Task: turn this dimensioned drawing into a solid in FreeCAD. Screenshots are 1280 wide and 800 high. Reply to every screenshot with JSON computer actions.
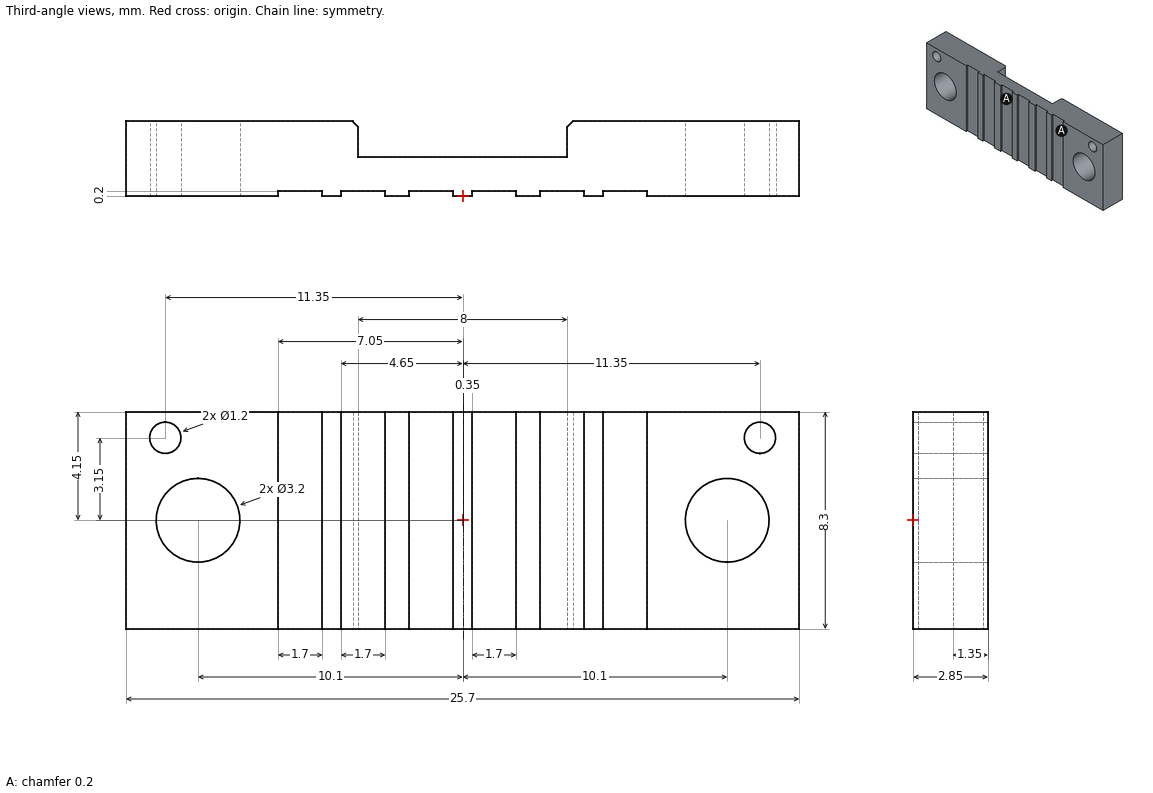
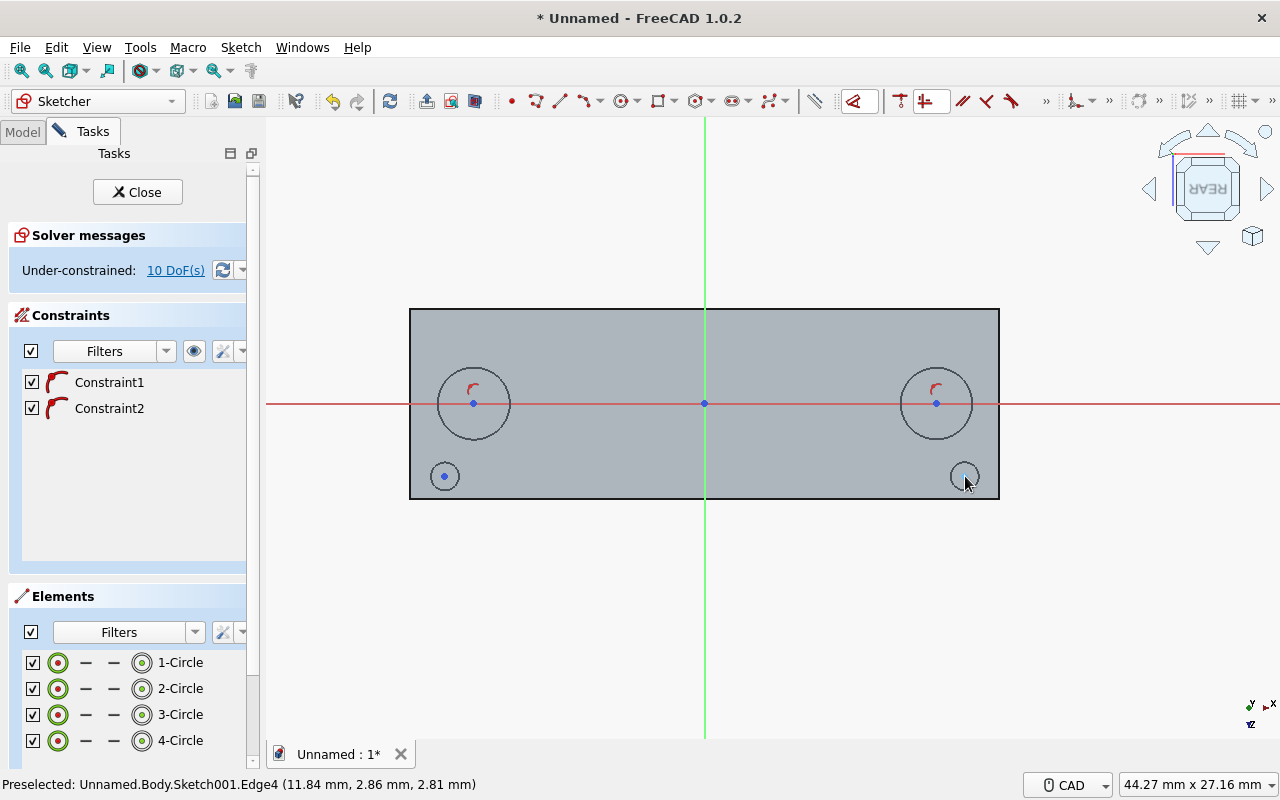
{"action": "left_click", "coordinate": [499, 378]}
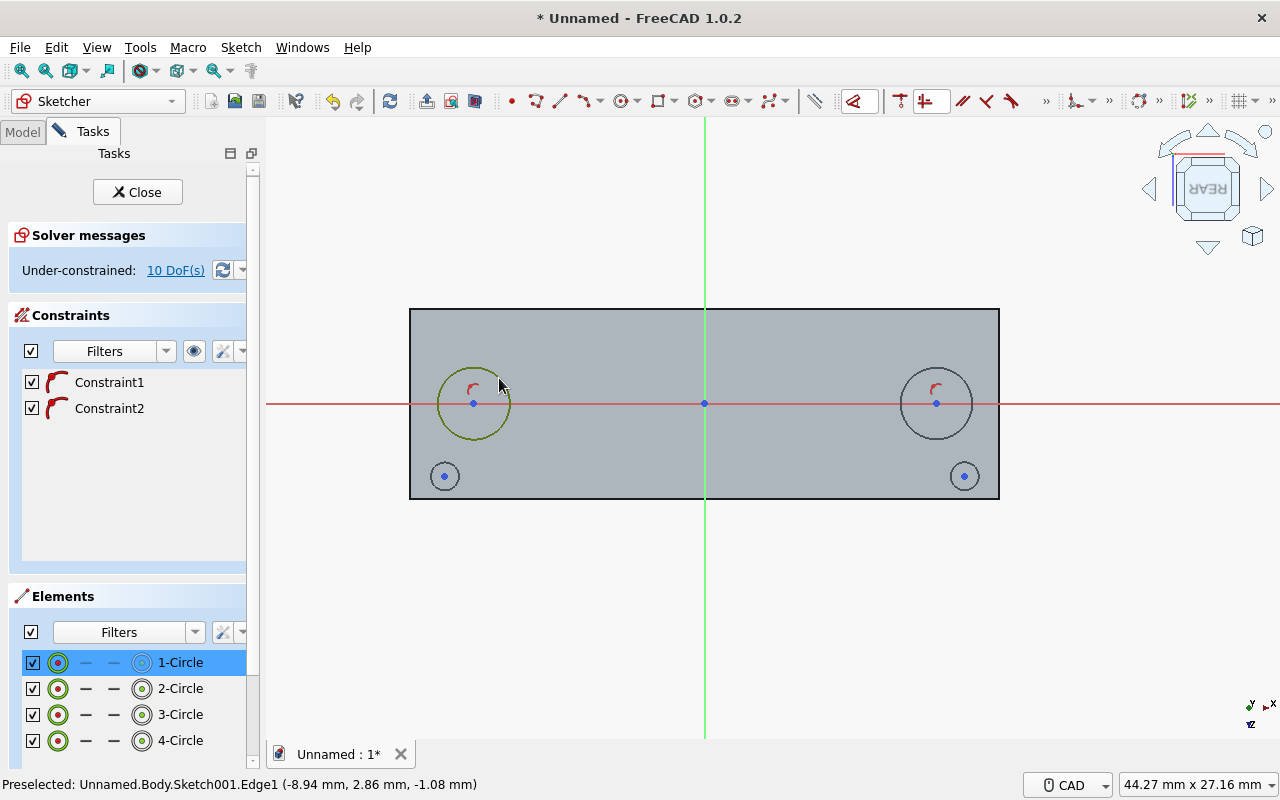
{"action": "left_click", "coordinate": [962, 378]}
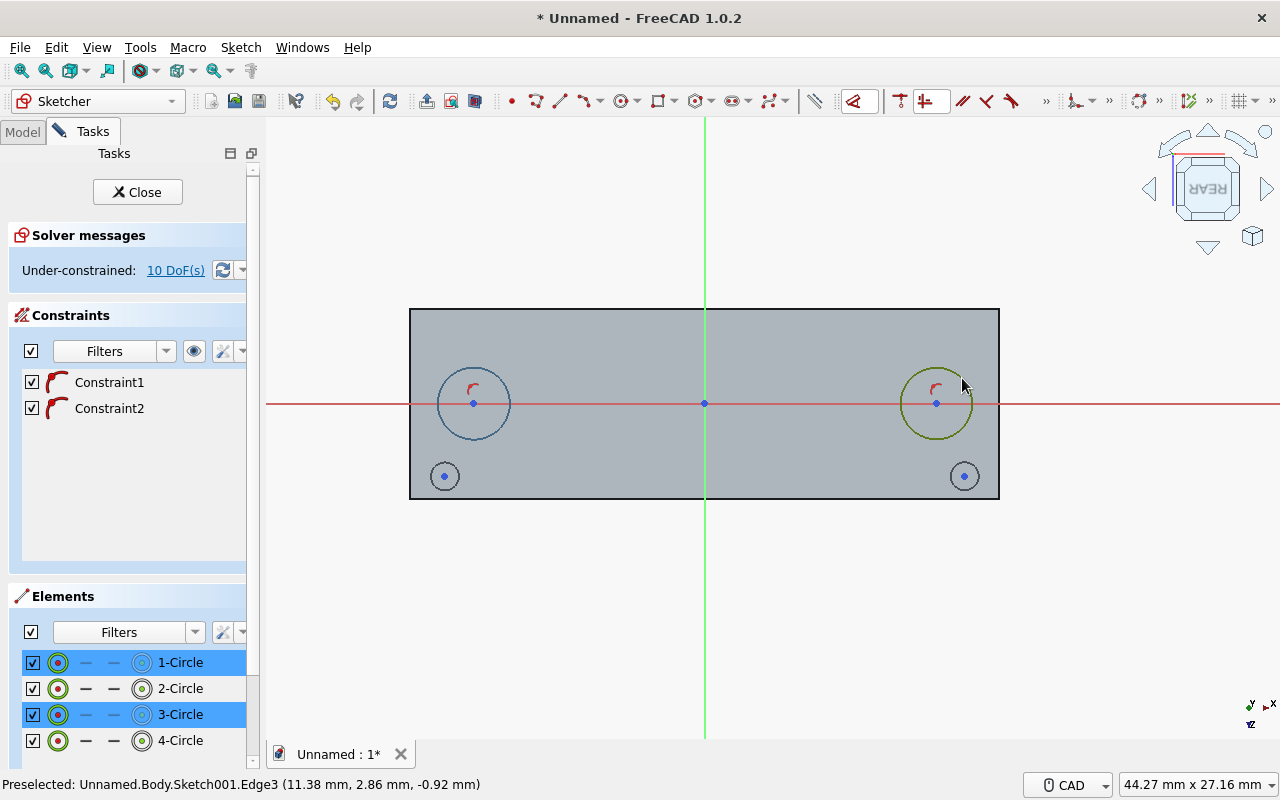
{"action": "key", "text": "e"}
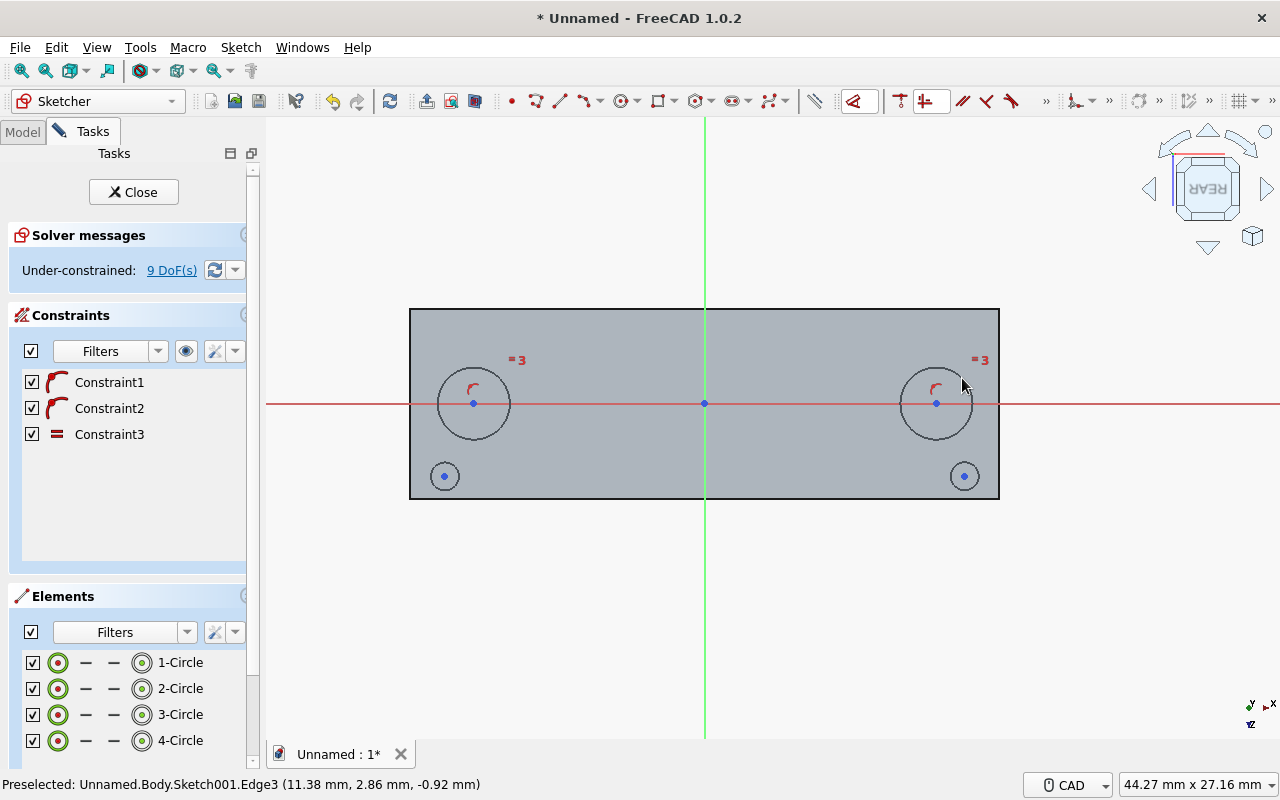
{"action": "left_click", "coordinate": [455, 467]}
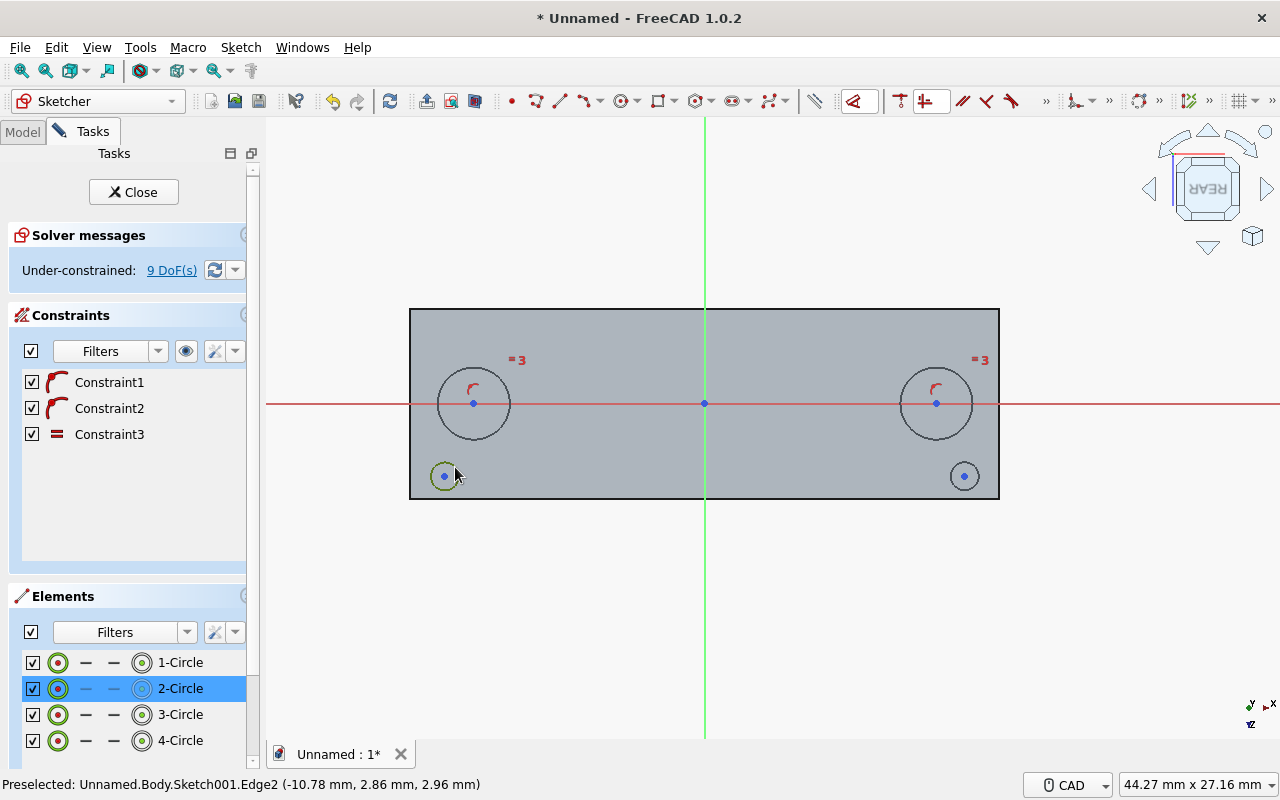
{"action": "left_click", "coordinate": [975, 466]}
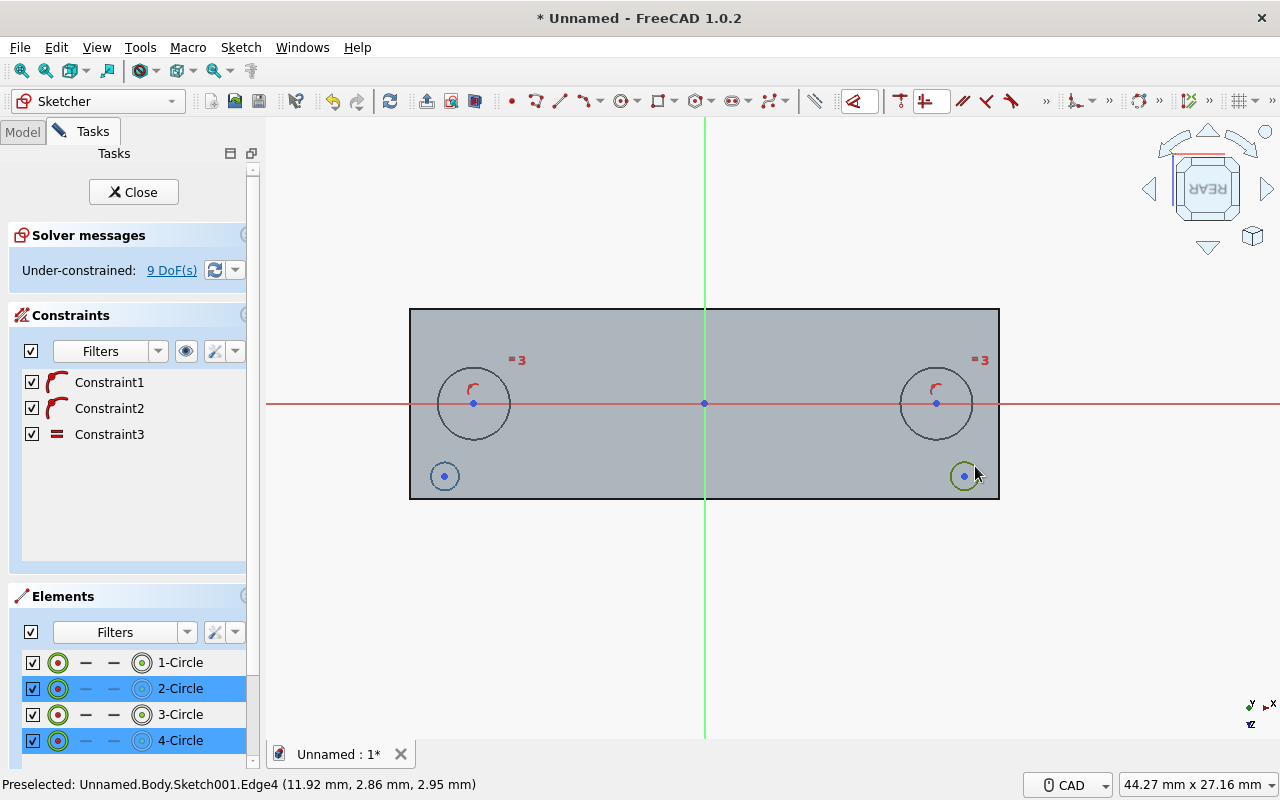
{"action": "key", "text": "e"}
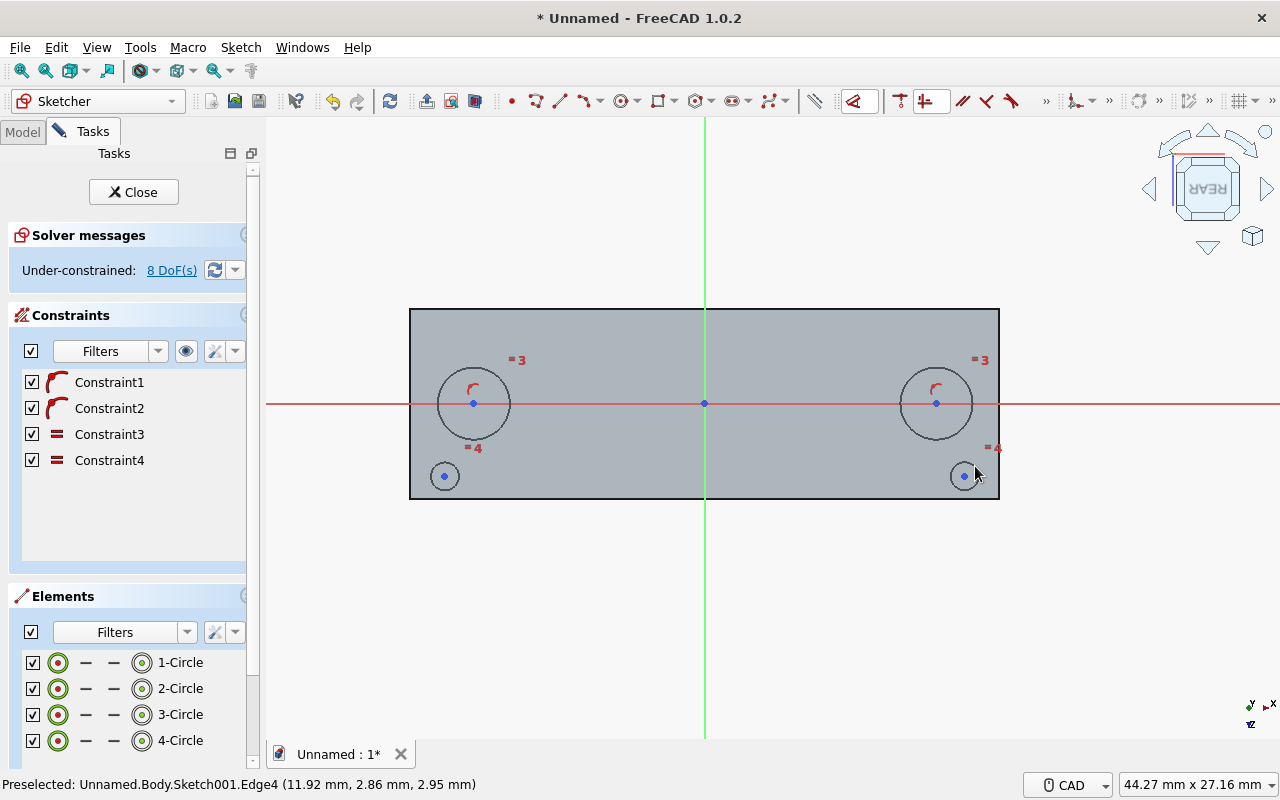
{"action": "left_click", "coordinate": [445, 476]}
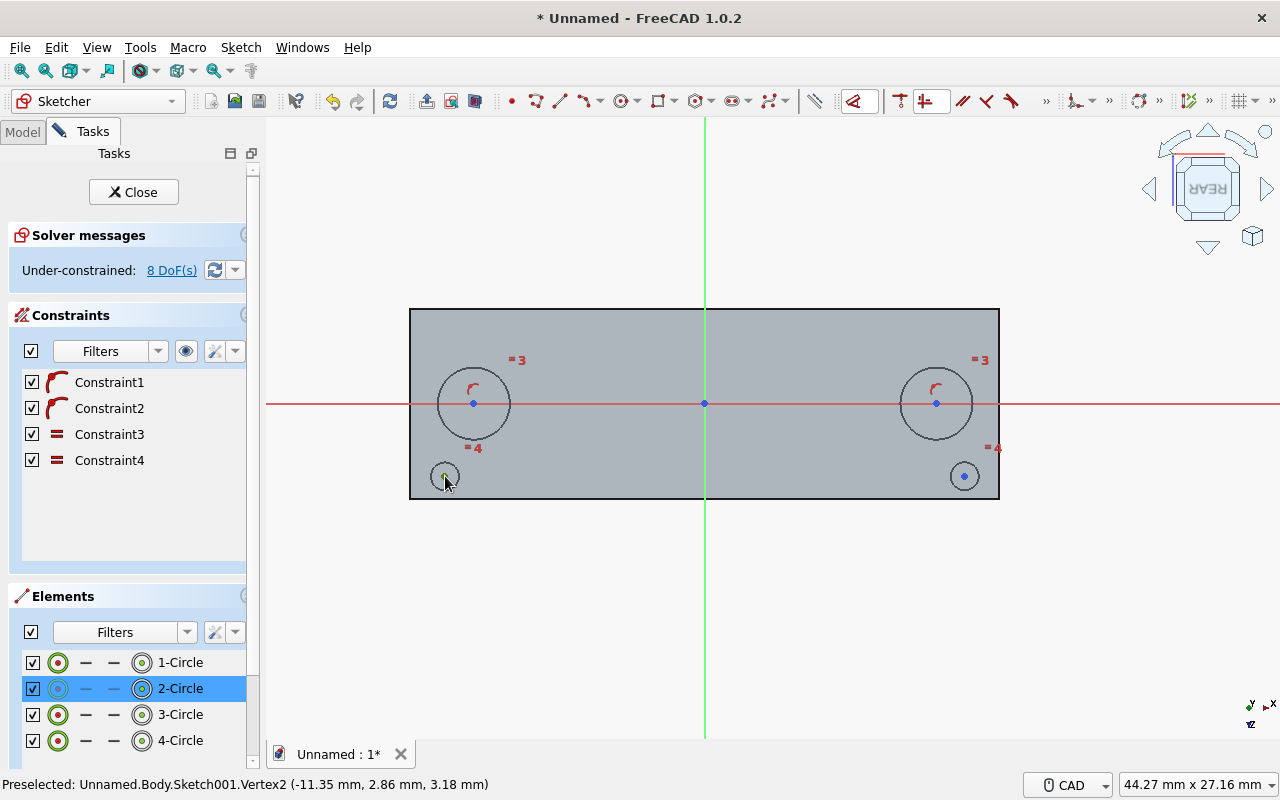
{"action": "left_click", "coordinate": [965, 476]}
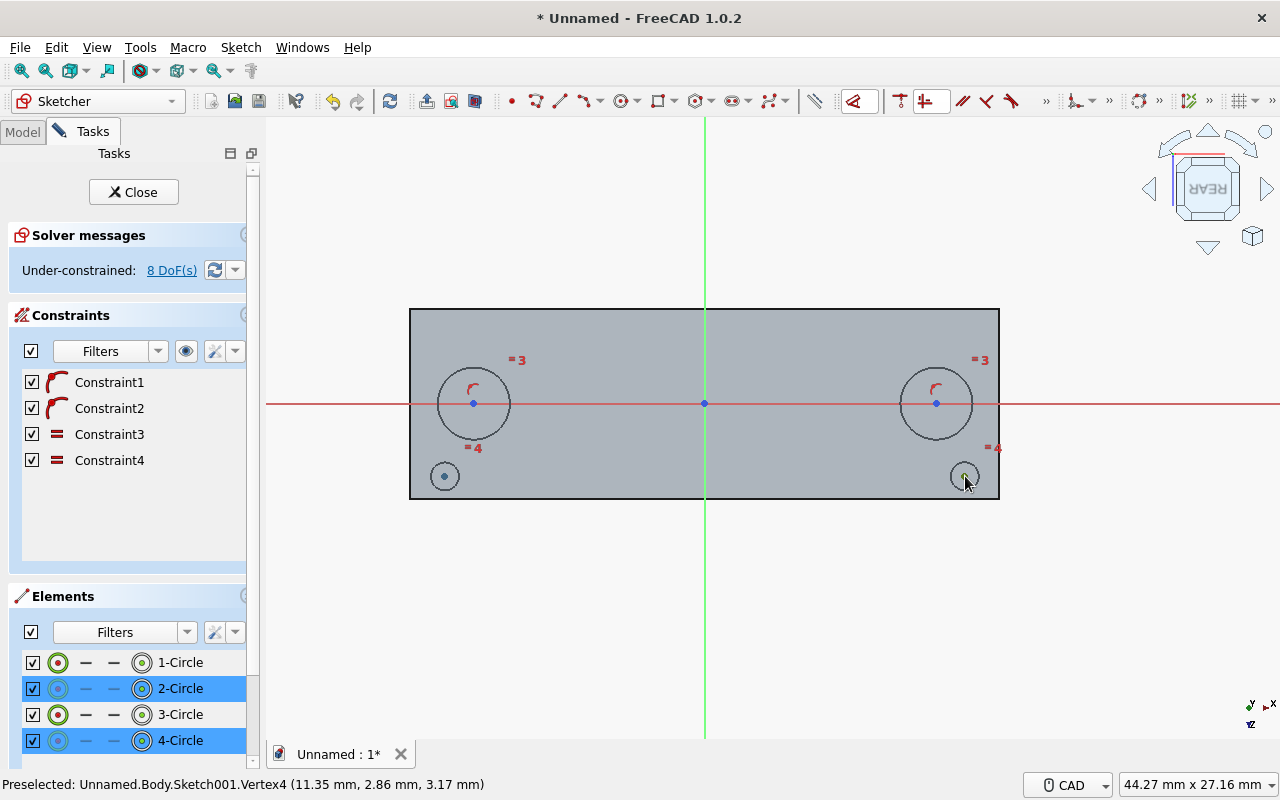
{"action": "key", "text": "h"}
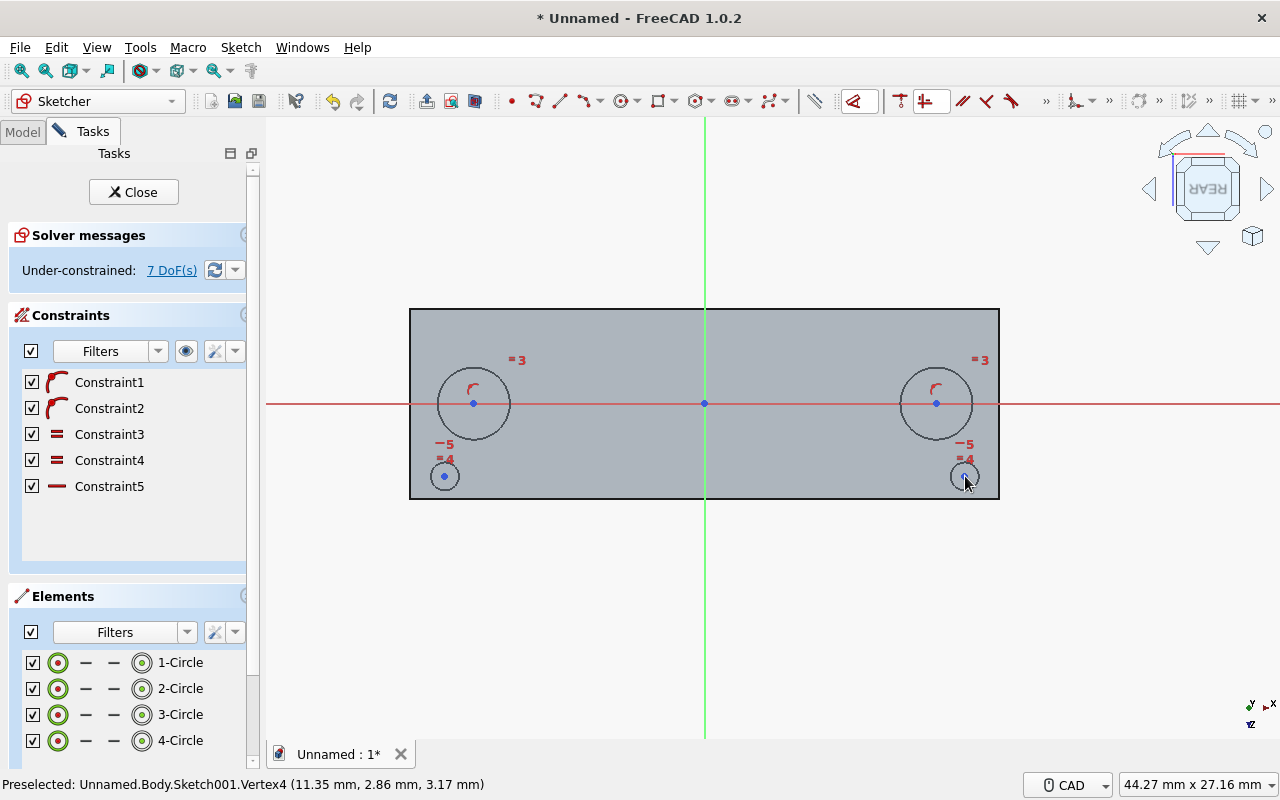
{"action": "key", "text": "d"}